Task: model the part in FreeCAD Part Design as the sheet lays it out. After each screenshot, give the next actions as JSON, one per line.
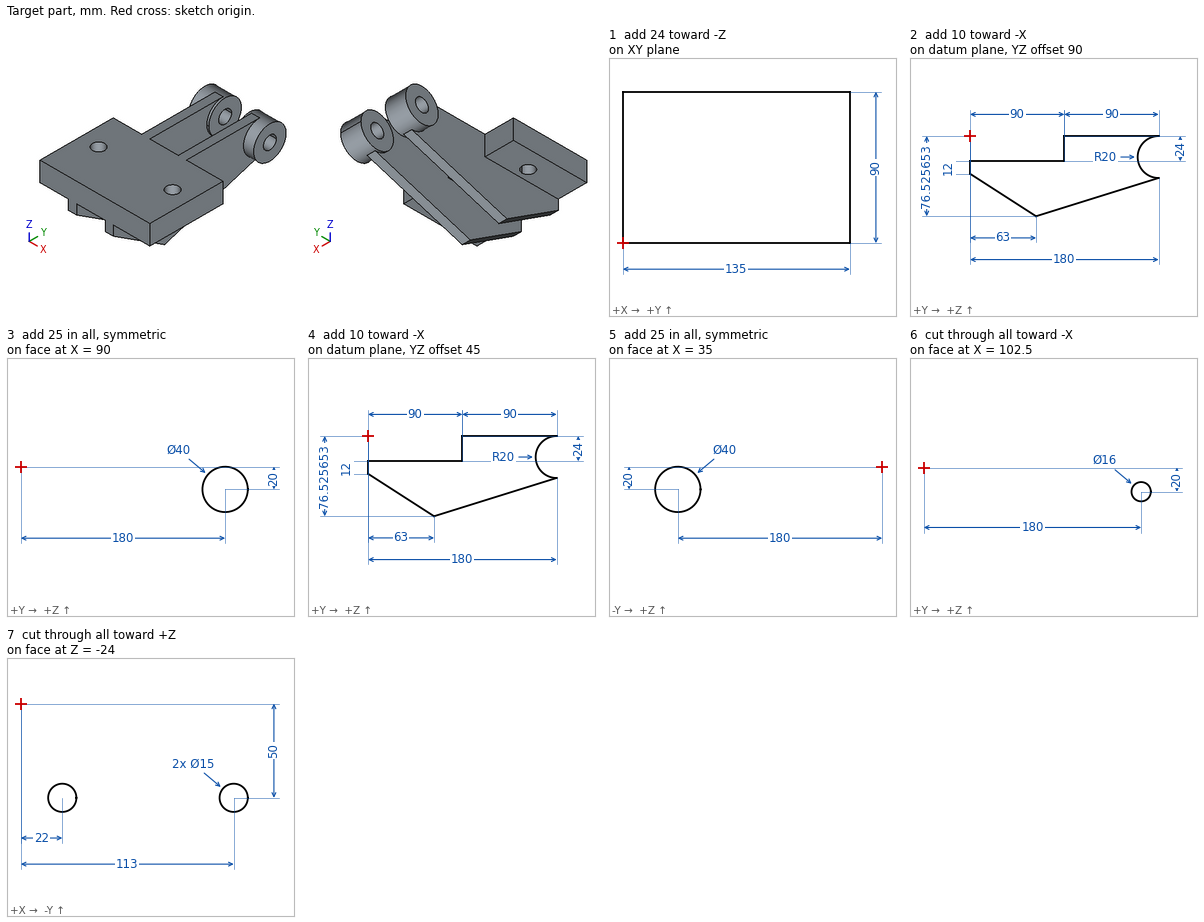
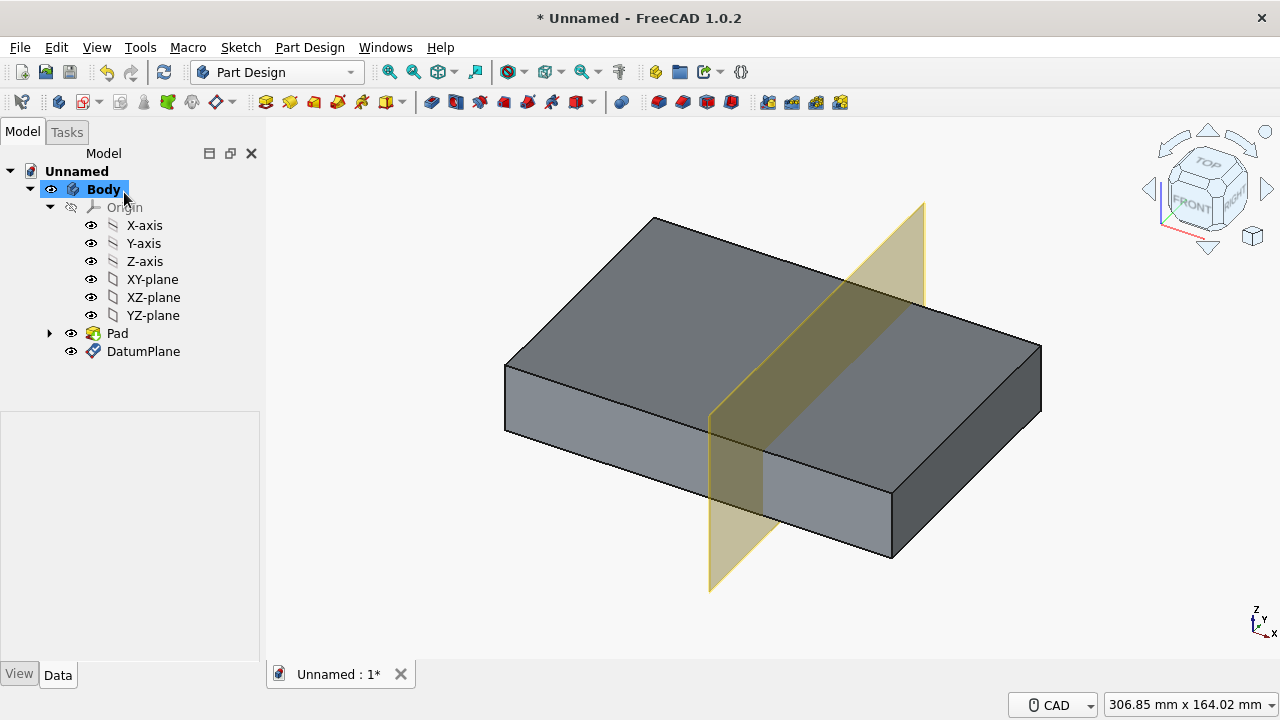
{"action": "left_click", "coordinate": [116, 351]}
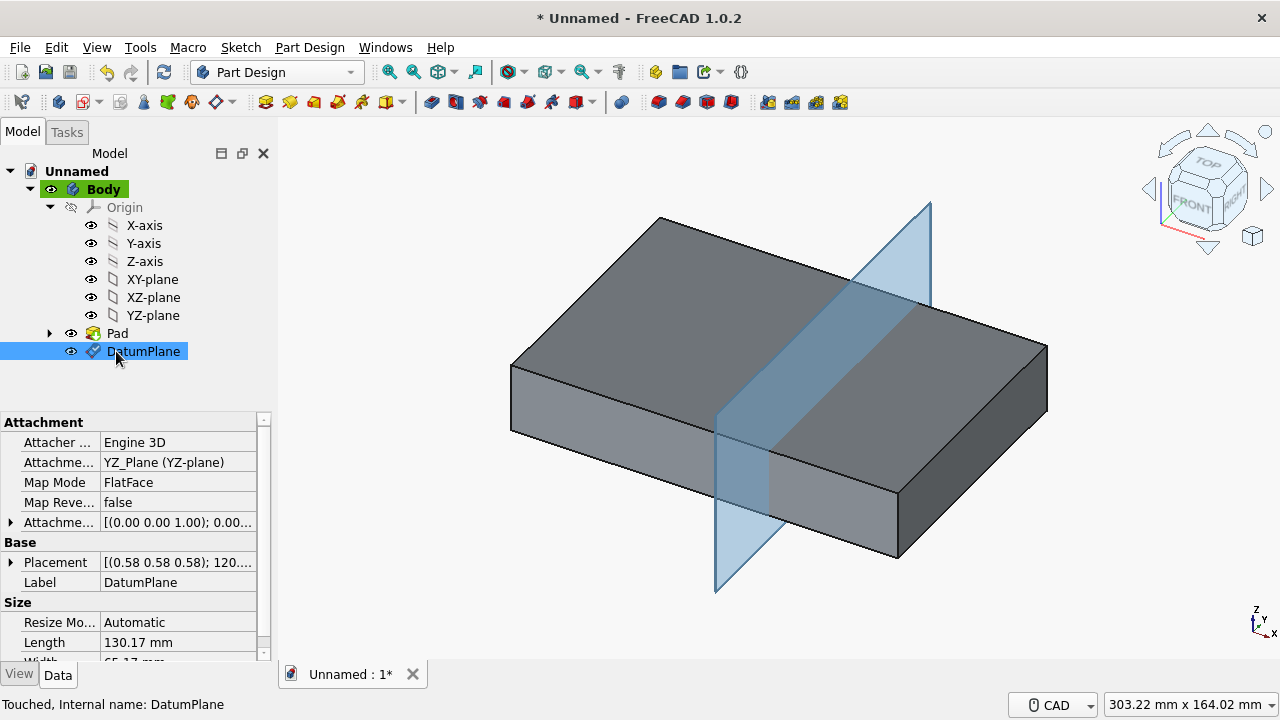
{"action": "left_click", "coordinate": [84, 102]}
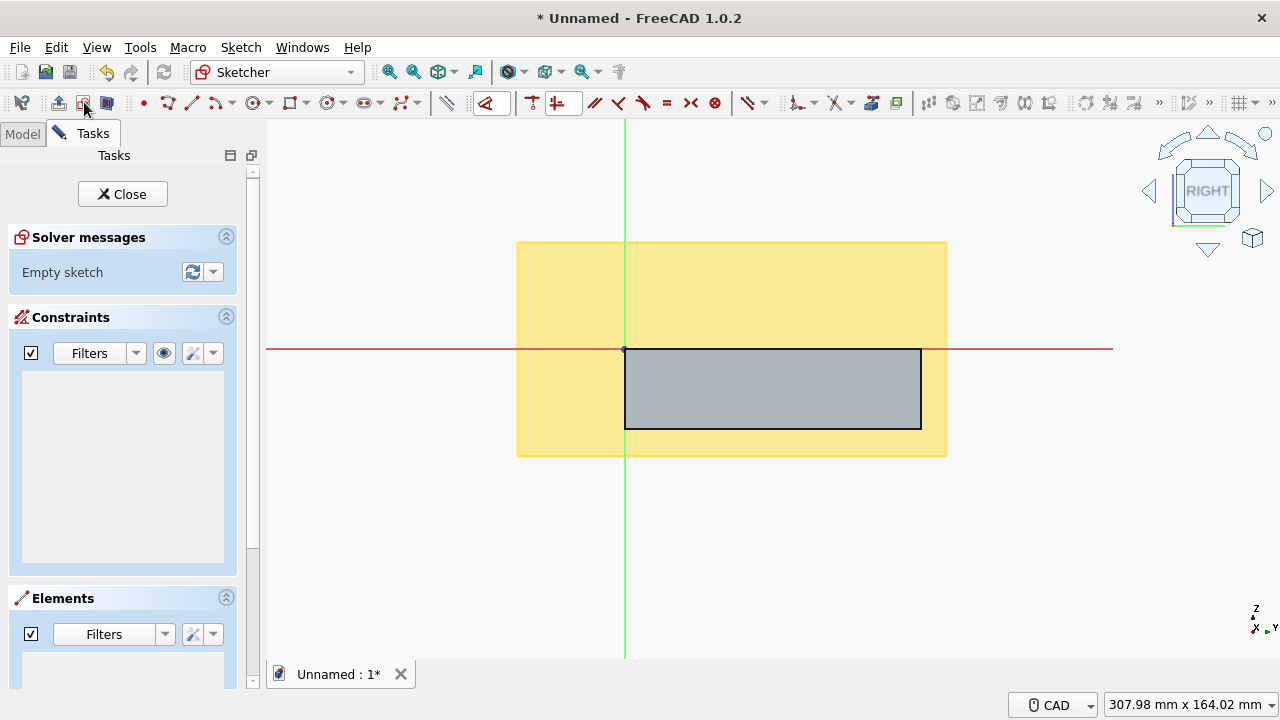
{"action": "left_click", "coordinate": [108, 104]}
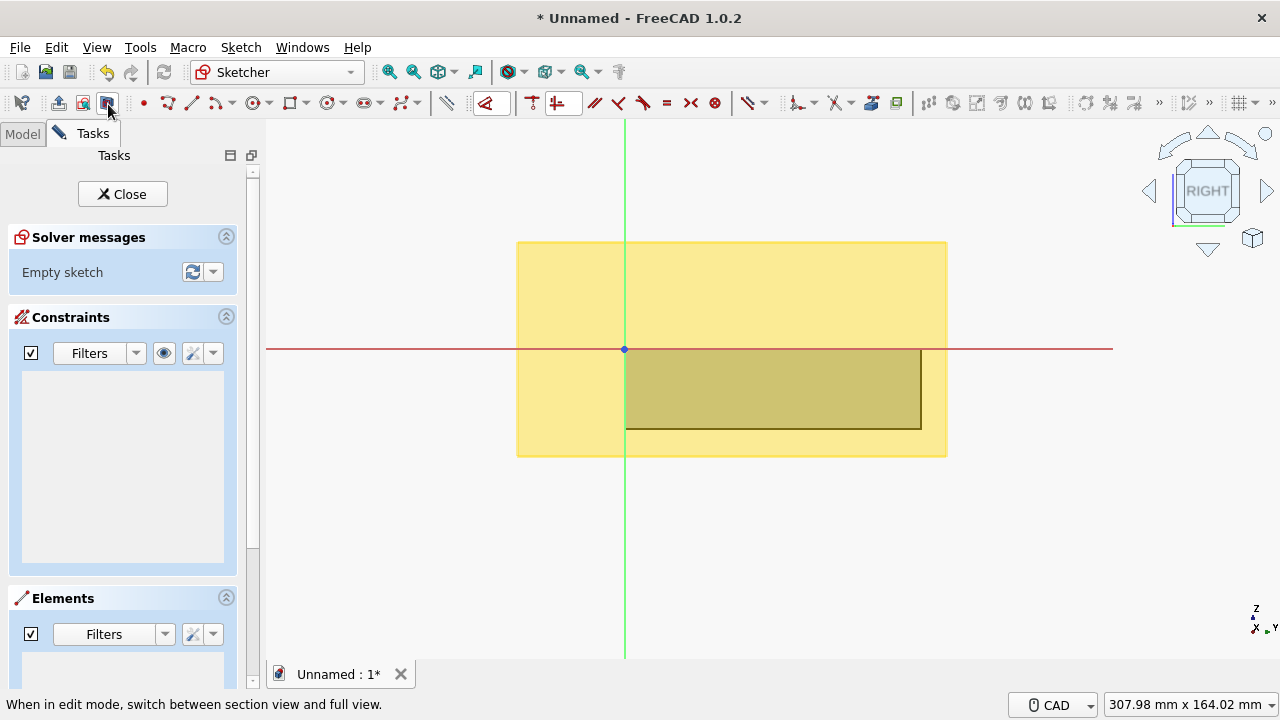
{"action": "scroll", "coordinate": [294, 147], "scroll_direction": "down", "scroll_amount": 1}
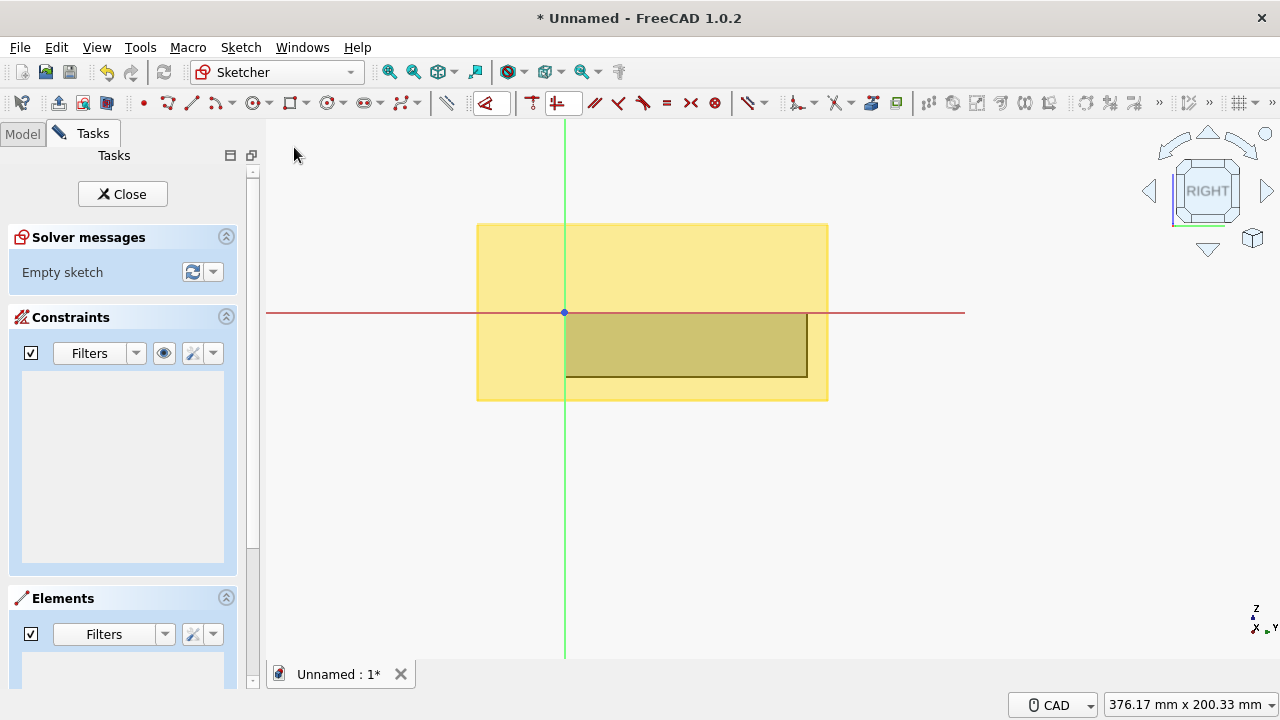
{"action": "key", "text": "g m"}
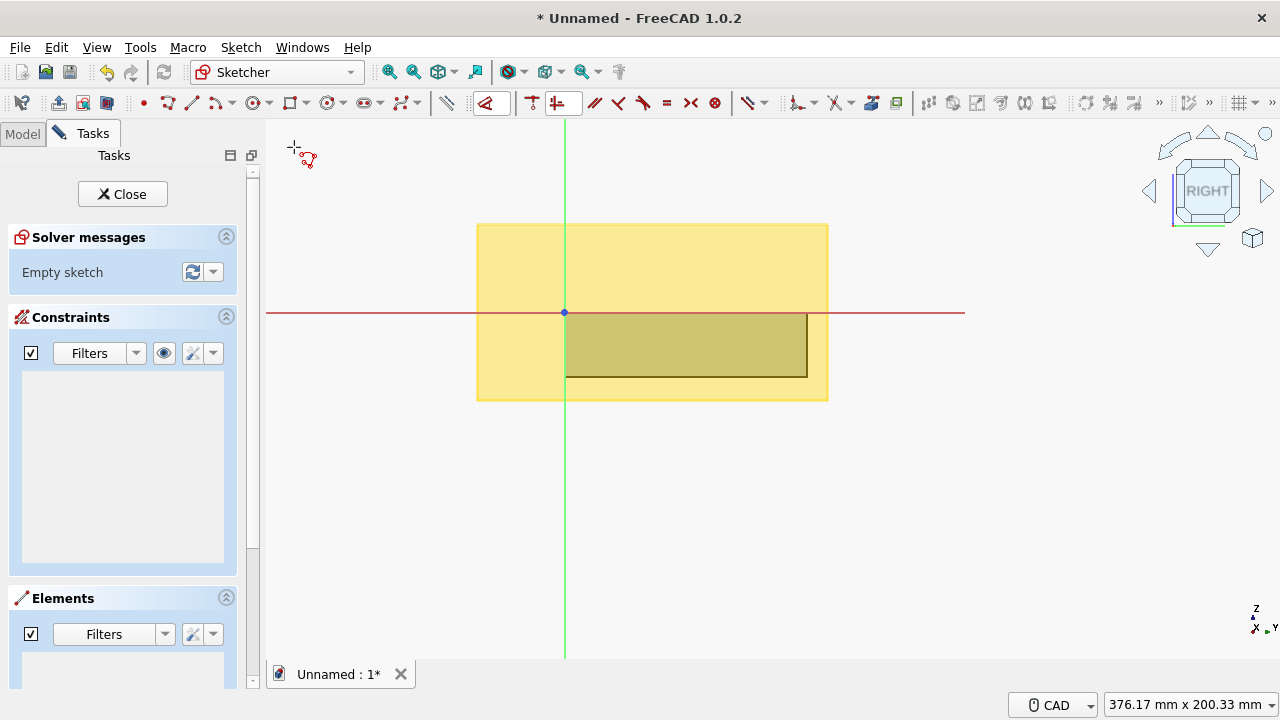
{"action": "left_click", "coordinate": [1050, 313]}
{"action": "left_click", "coordinate": [807, 322]}
{"action": "left_click", "coordinate": [807, 377]}
{"action": "left_click", "coordinate": [565, 377]}
{"action": "left_click", "coordinate": [574, 410]}
{"action": "left_click", "coordinate": [735, 519]}
{"action": "left_click", "coordinate": [1050, 421]}
{"action": "right_click", "coordinate": [1050, 421]}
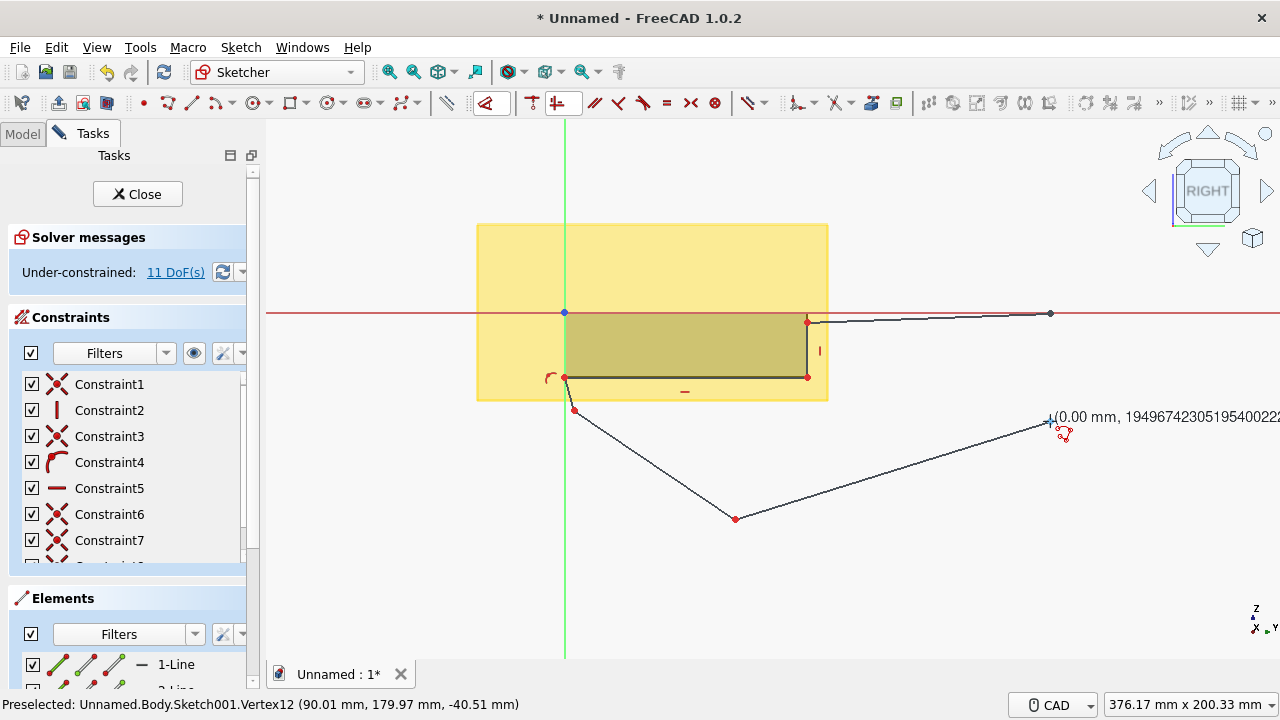
{"action": "key", "text": "g 3 a"}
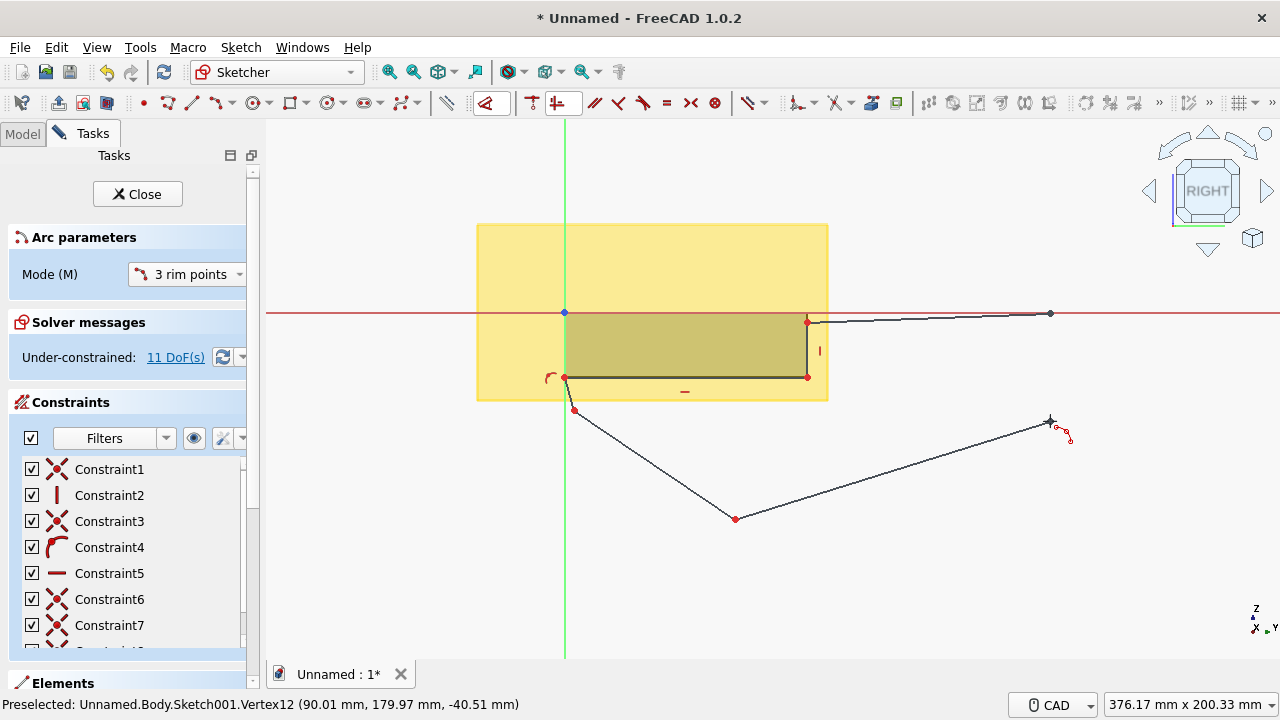
{"action": "left_click", "coordinate": [1050, 422]}
{"action": "left_click", "coordinate": [1050, 314]}
{"action": "left_click", "coordinate": [996, 367]}
{"action": "key", "text": "Escape"}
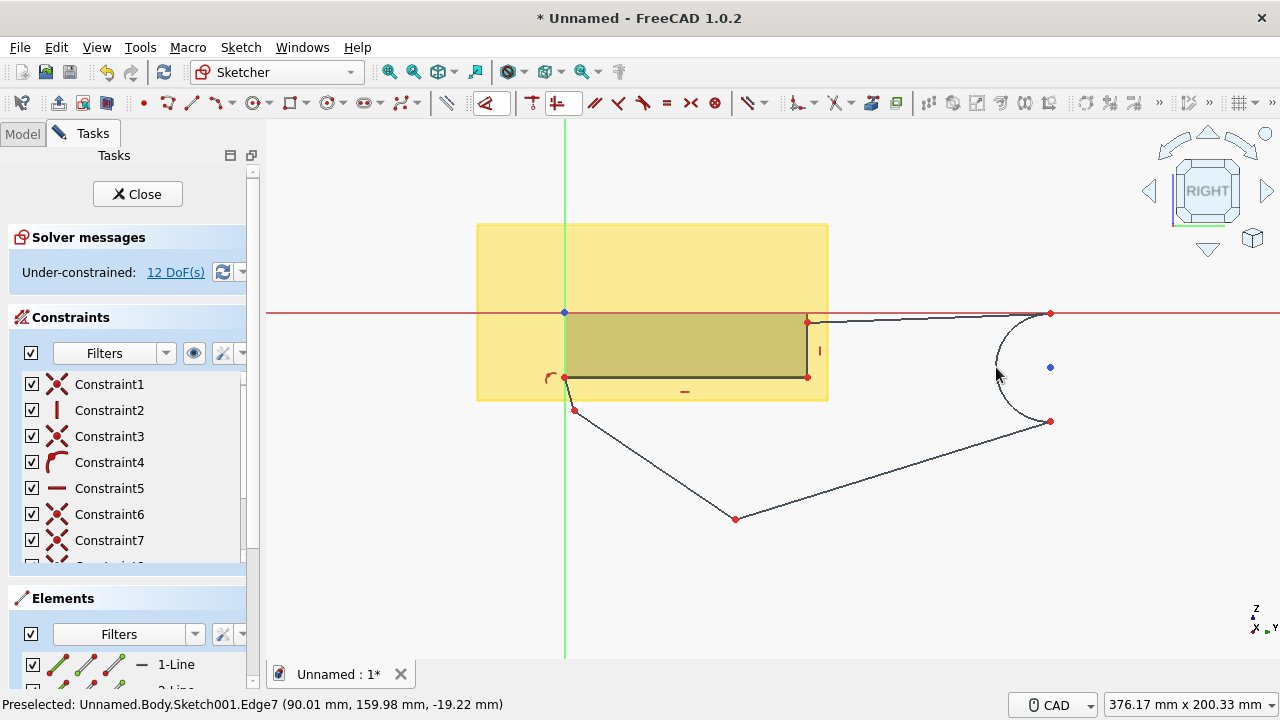
{"action": "left_click", "coordinate": [977, 317]}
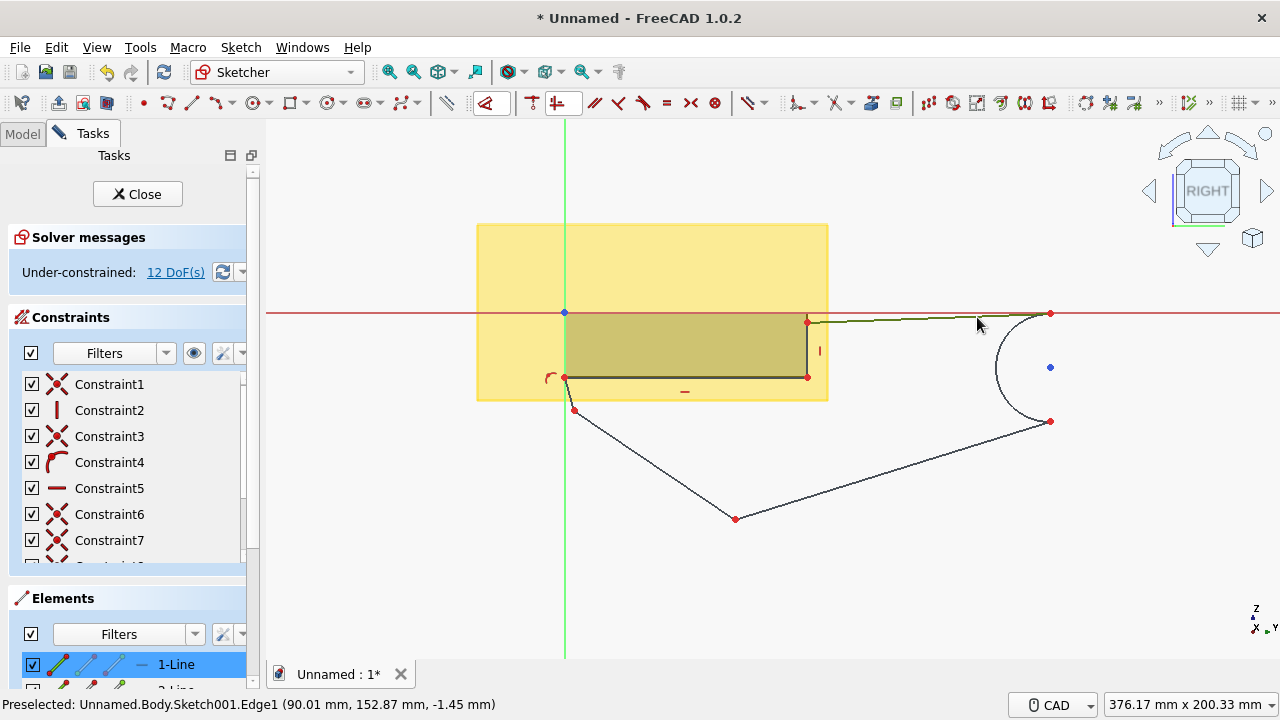
{"action": "left_click", "coordinate": [1006, 336]}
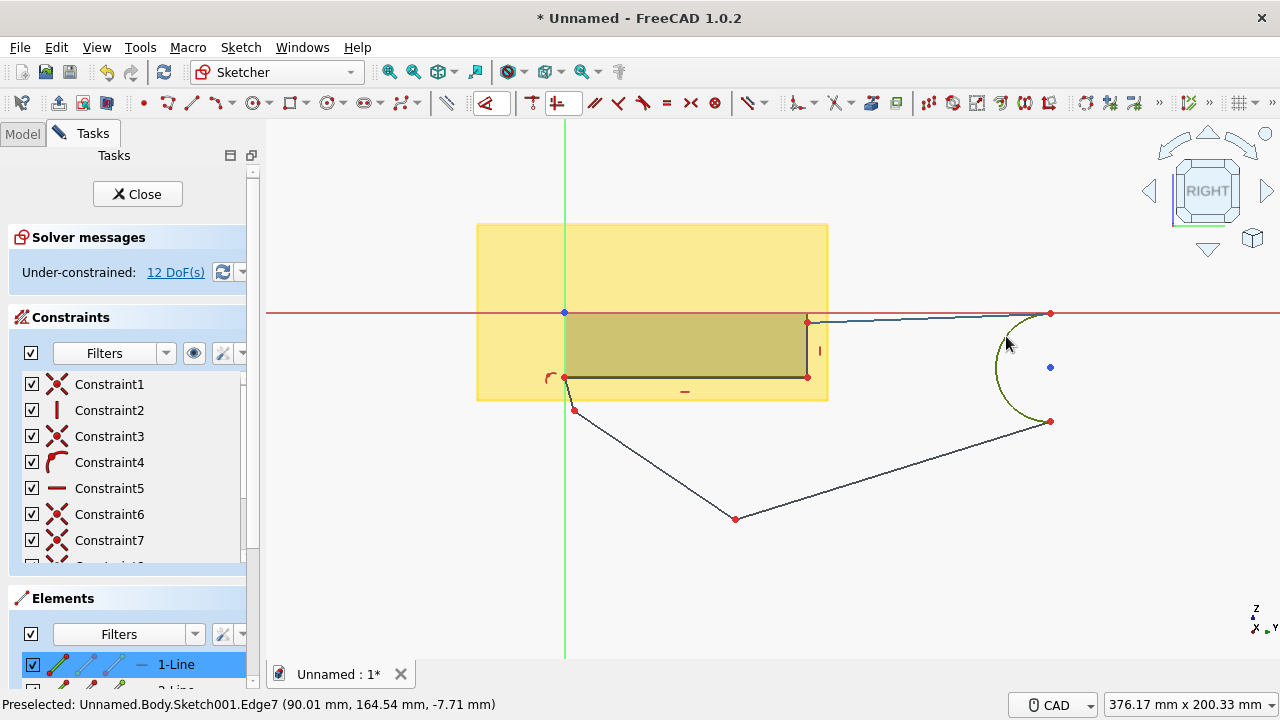
{"action": "left_click", "coordinate": [644, 104]}